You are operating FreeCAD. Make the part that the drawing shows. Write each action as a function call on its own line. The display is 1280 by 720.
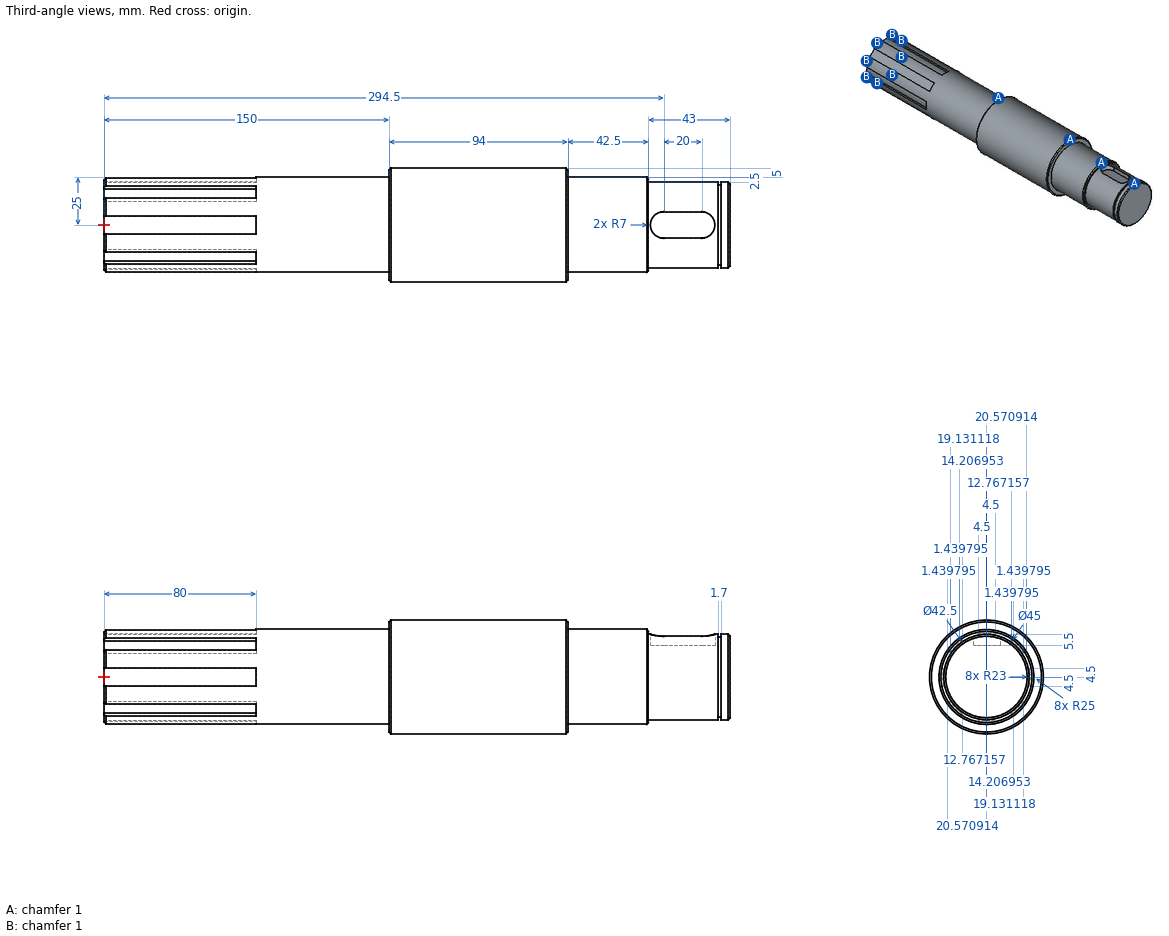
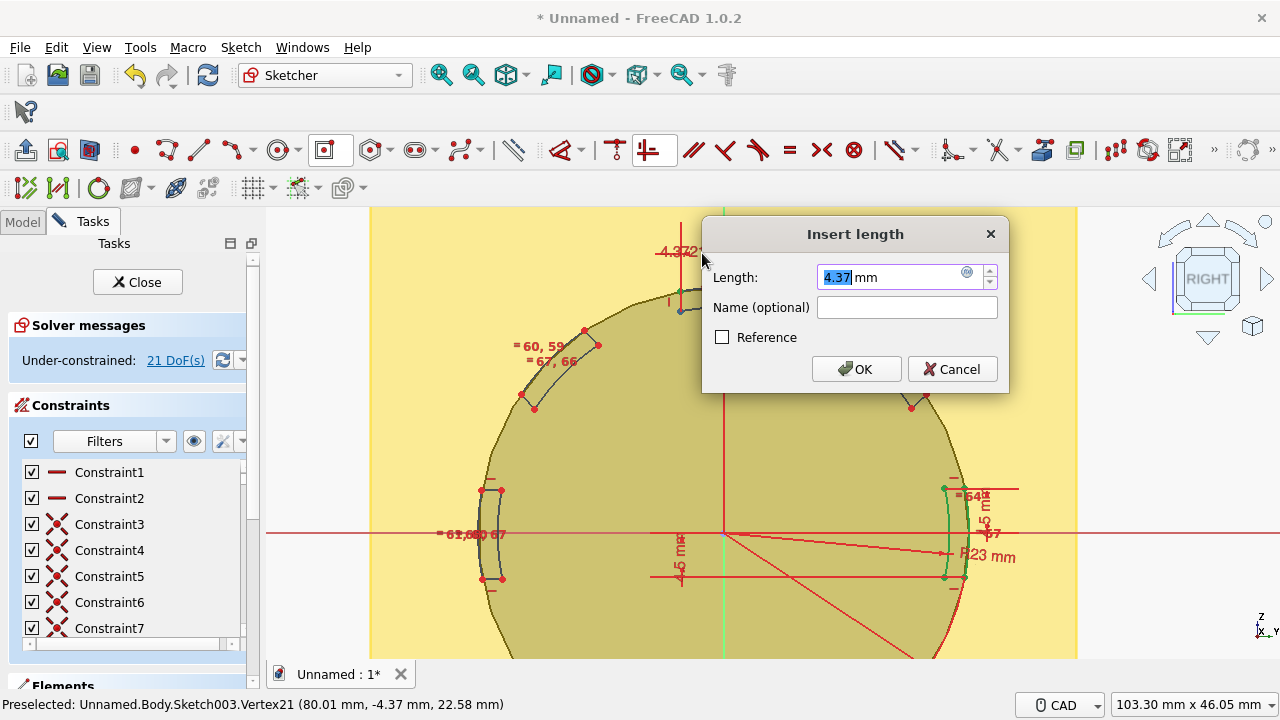
text(4.5)
key(Return)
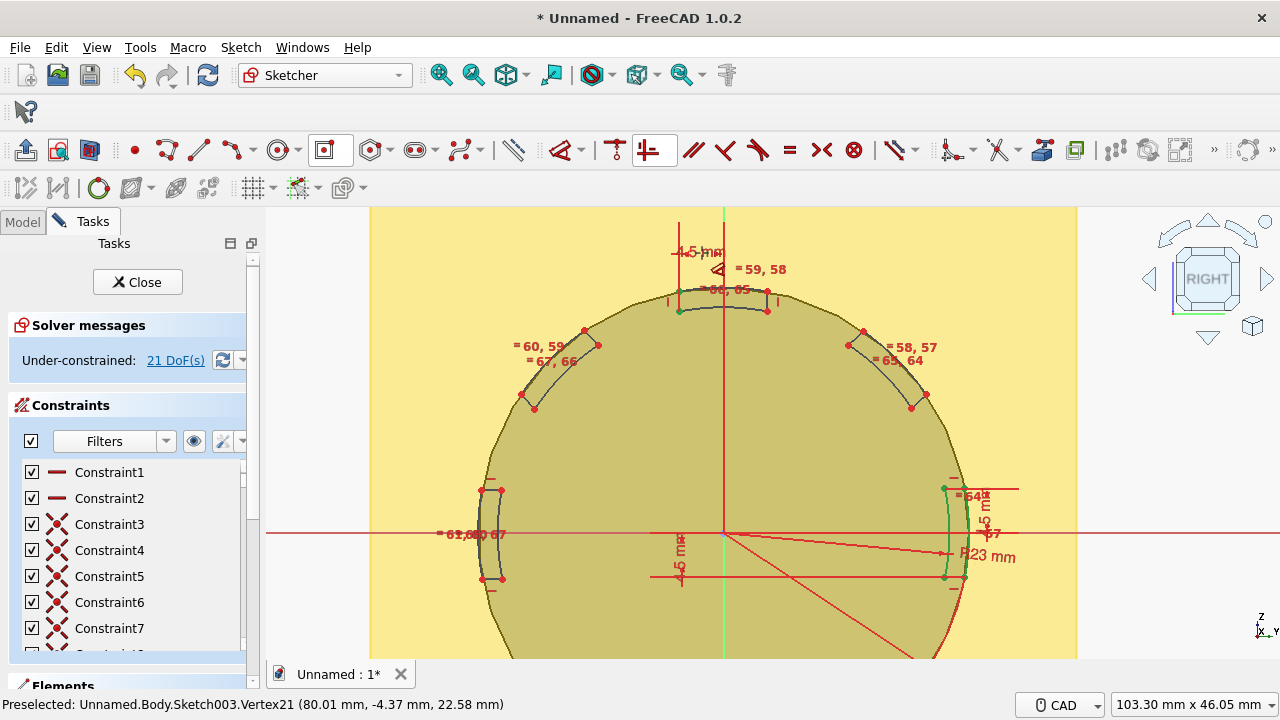
click(767, 292)
click(756, 567)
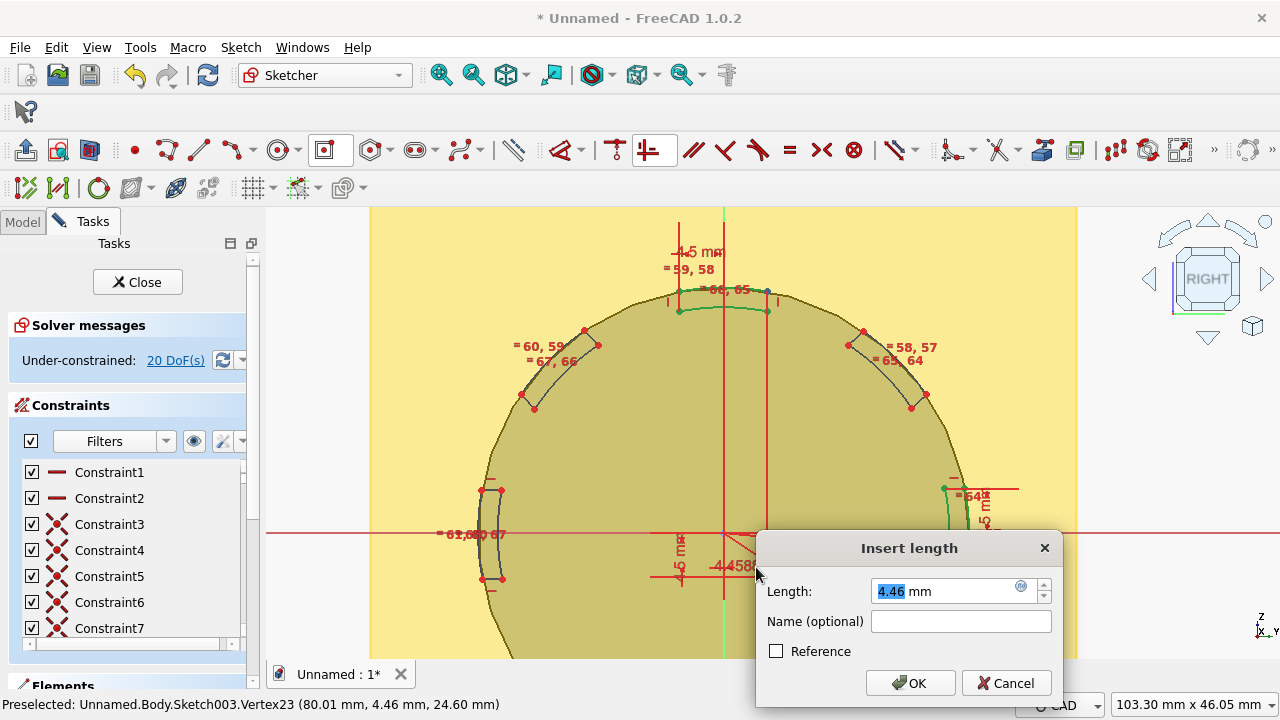
text(4.5)
key(Return)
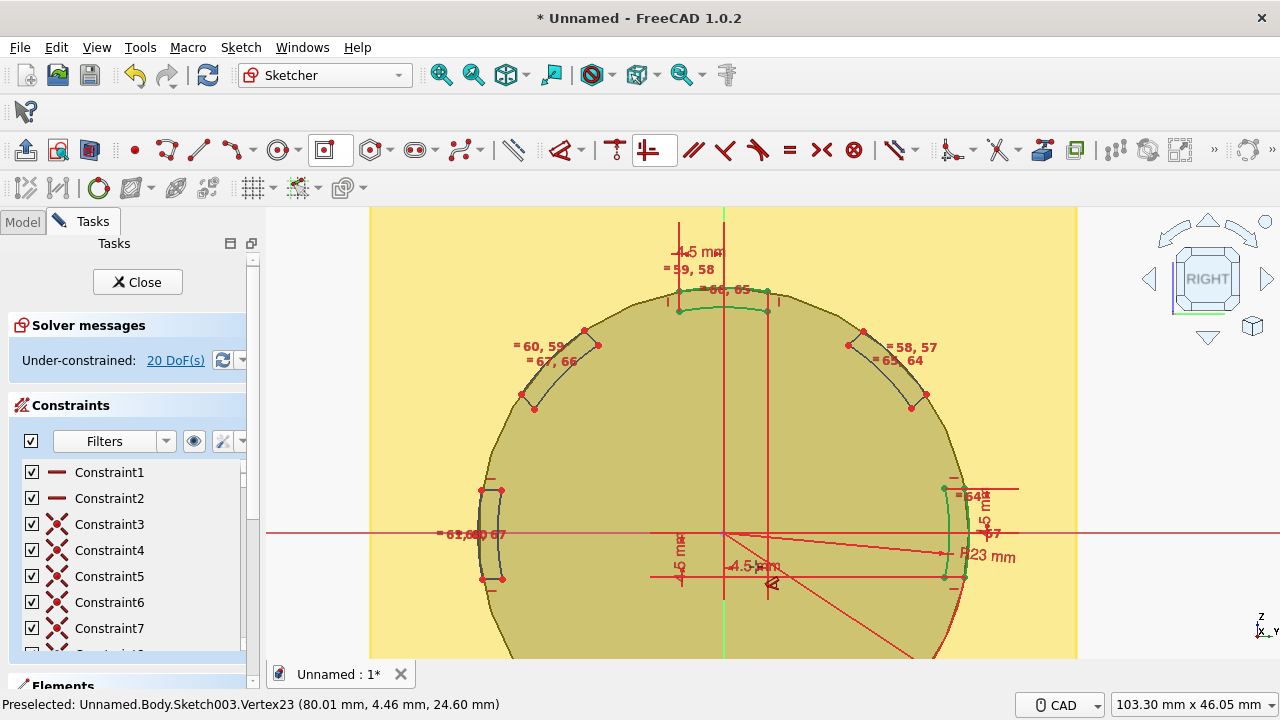
click(503, 579)
click(445, 556)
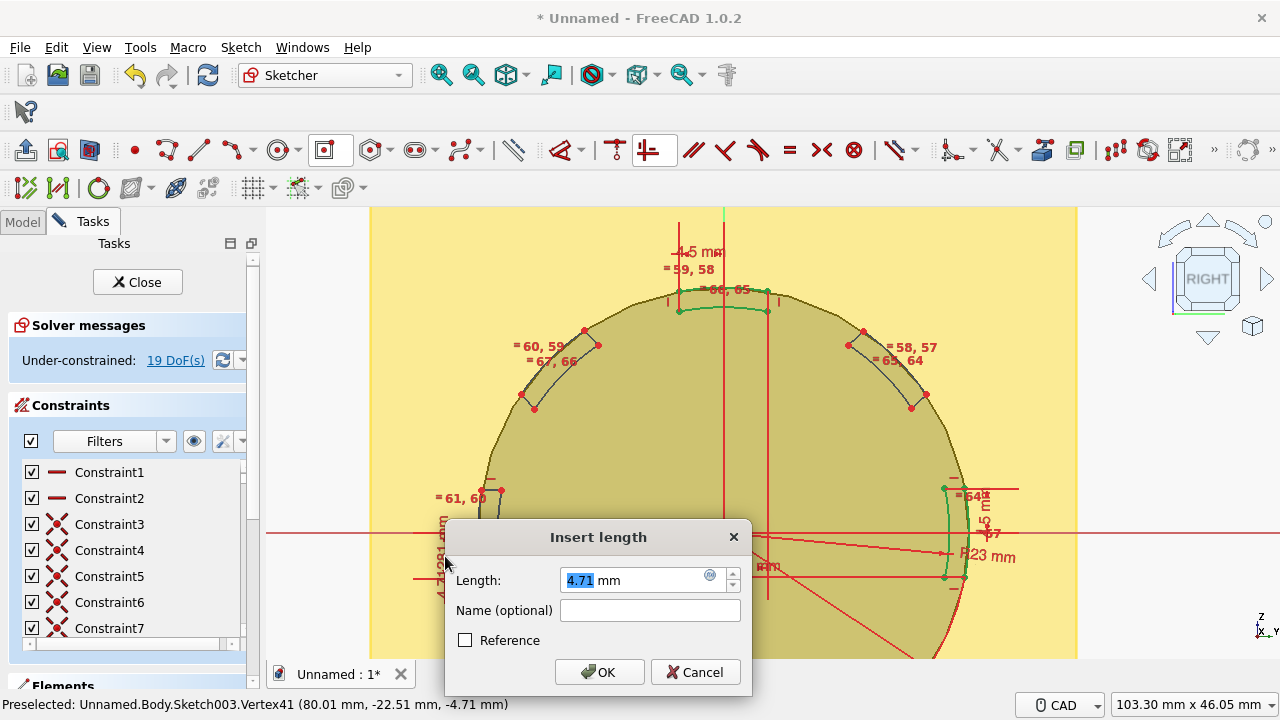
text(4.5)
key(Return)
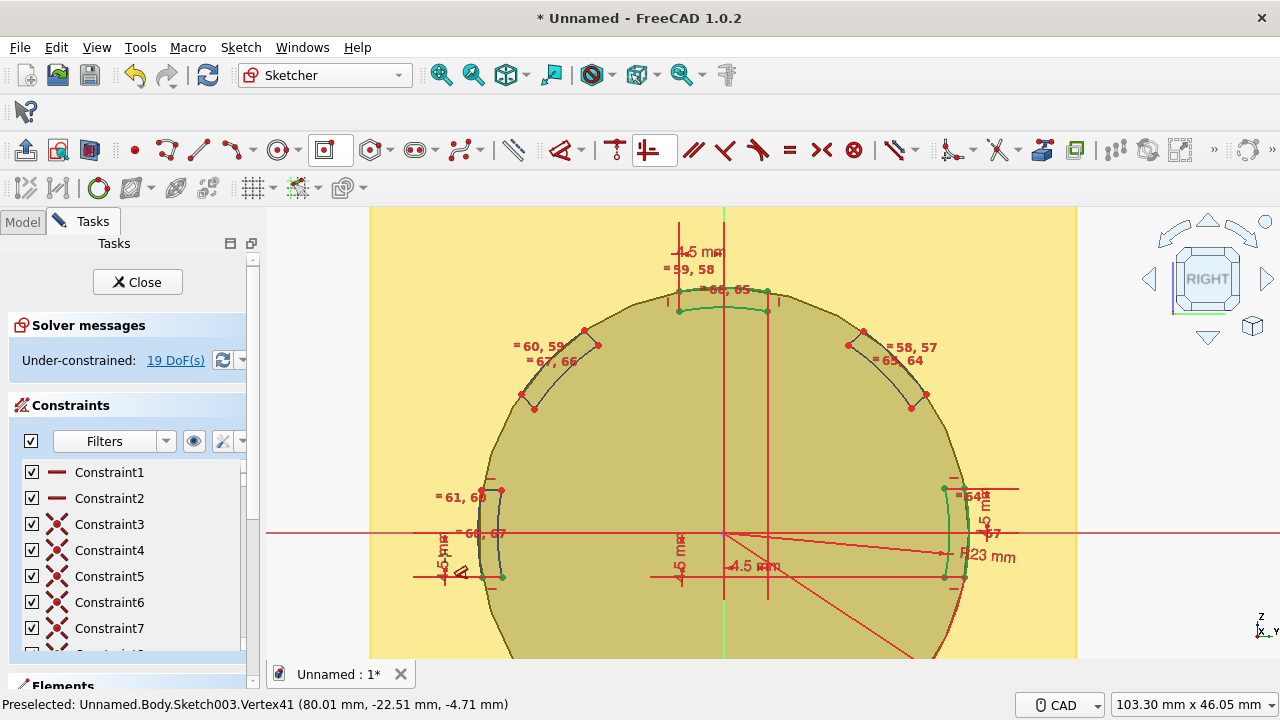
click(482, 490)
click(448, 512)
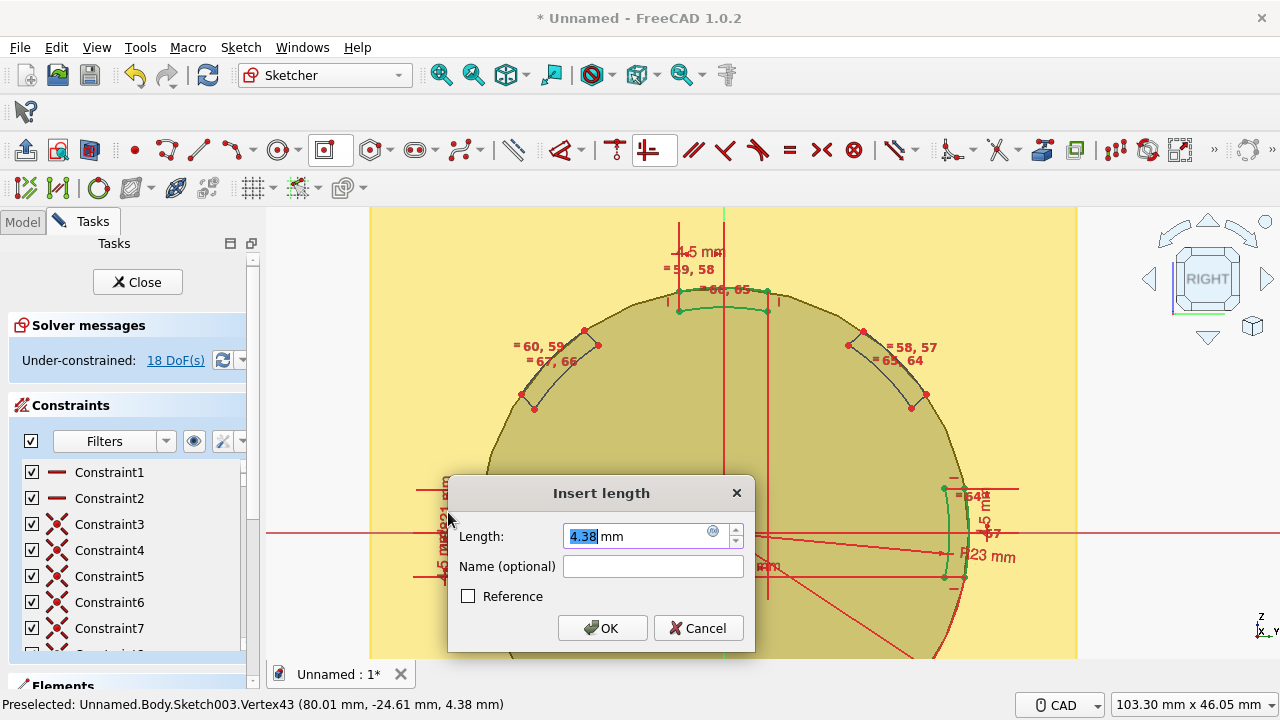
text(4.5)
key(Return)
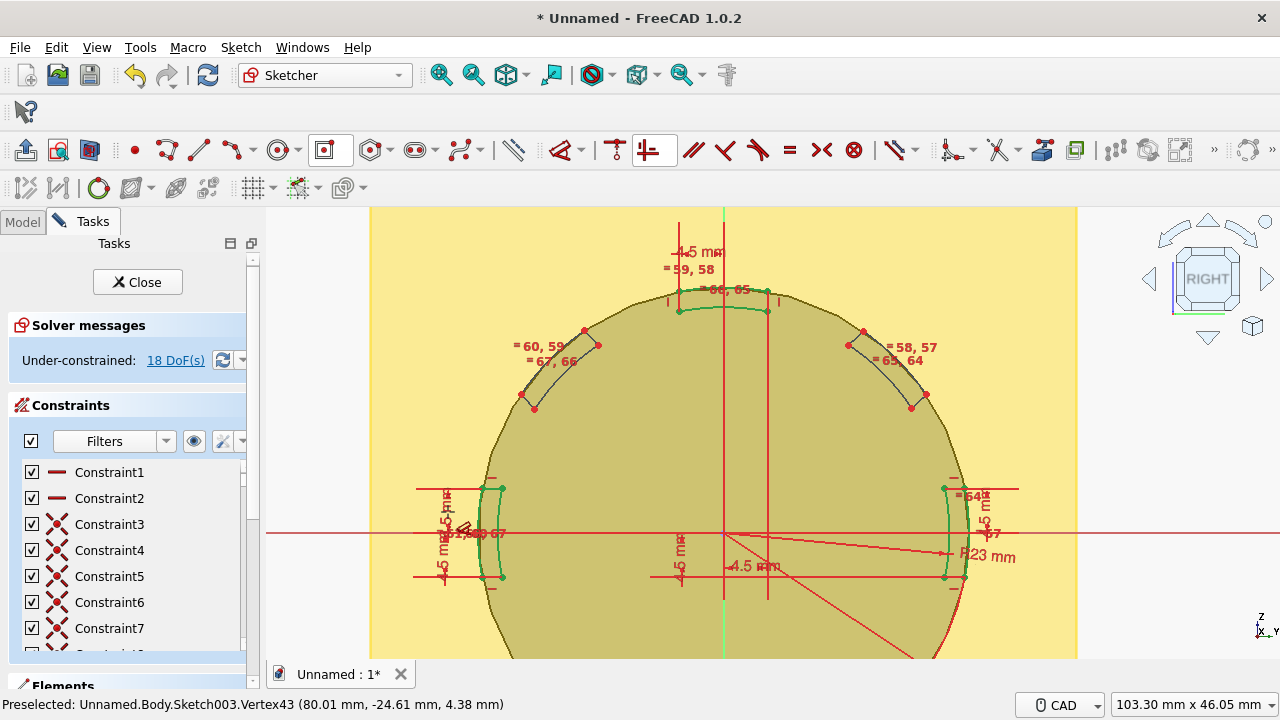
scroll(681, 311, down, 3)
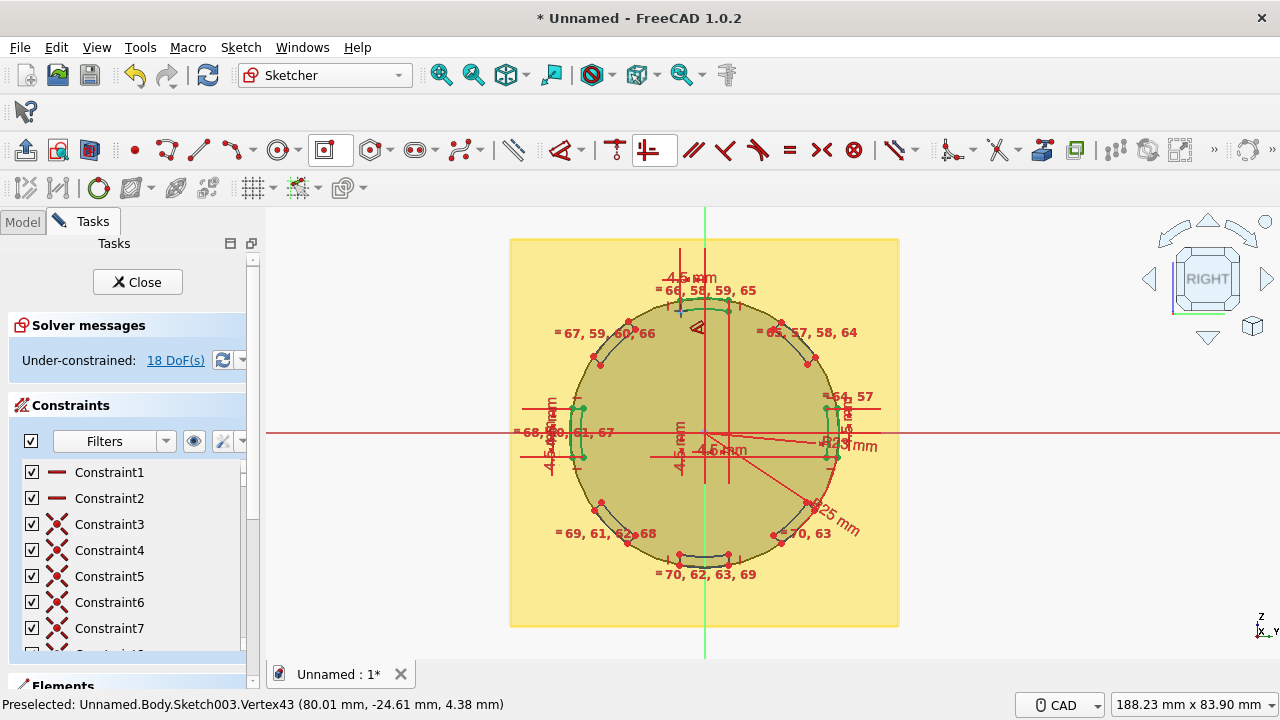
scroll(729, 554, up, 3)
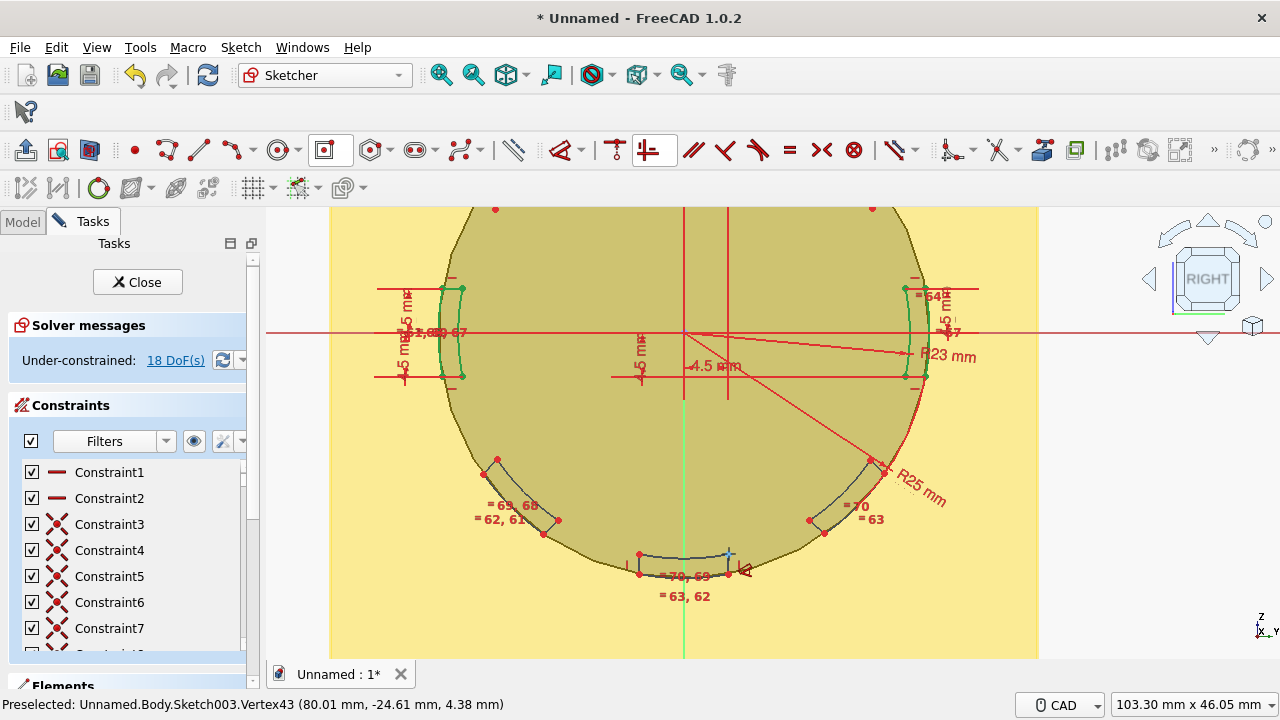
click(728, 554)
click(706, 299)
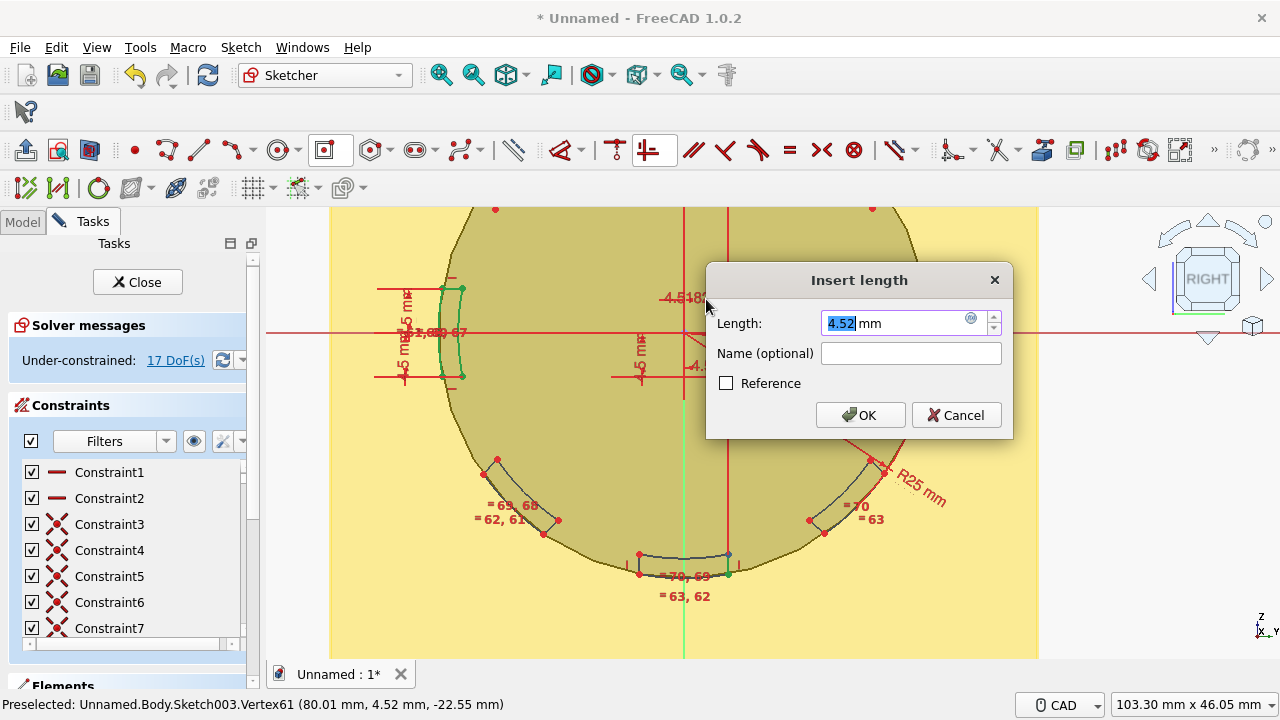
text(4.5)
key(Return)